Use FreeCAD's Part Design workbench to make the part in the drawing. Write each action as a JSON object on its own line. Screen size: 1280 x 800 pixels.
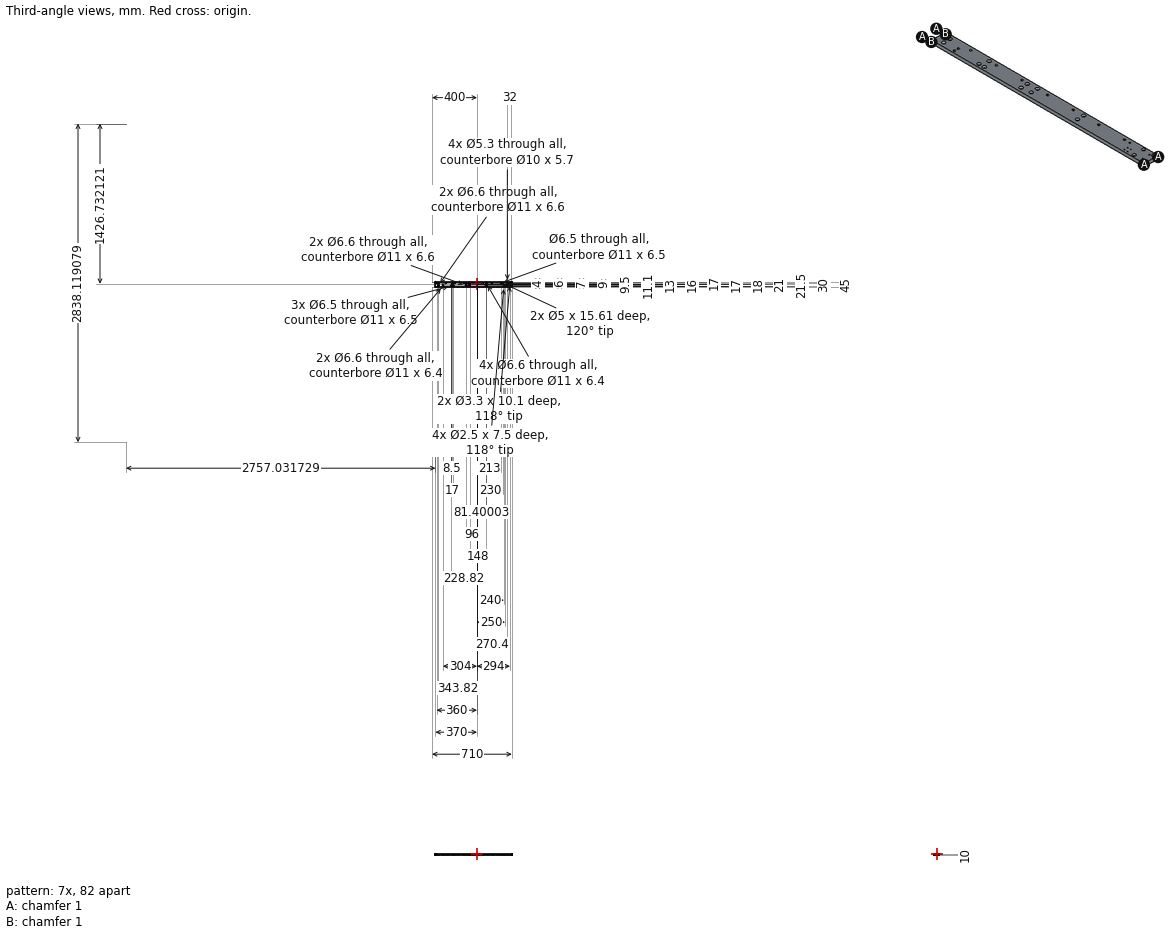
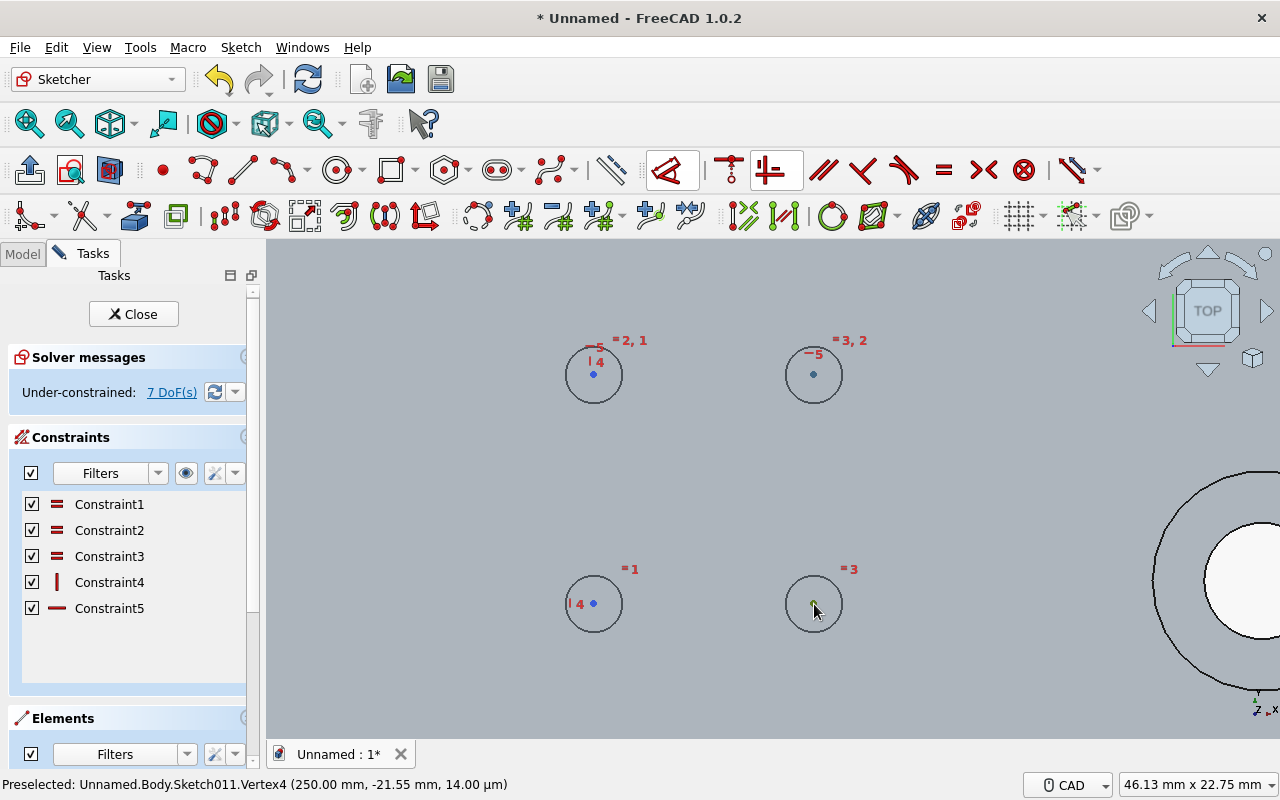
{"action": "left_click", "coordinate": [798, 170]}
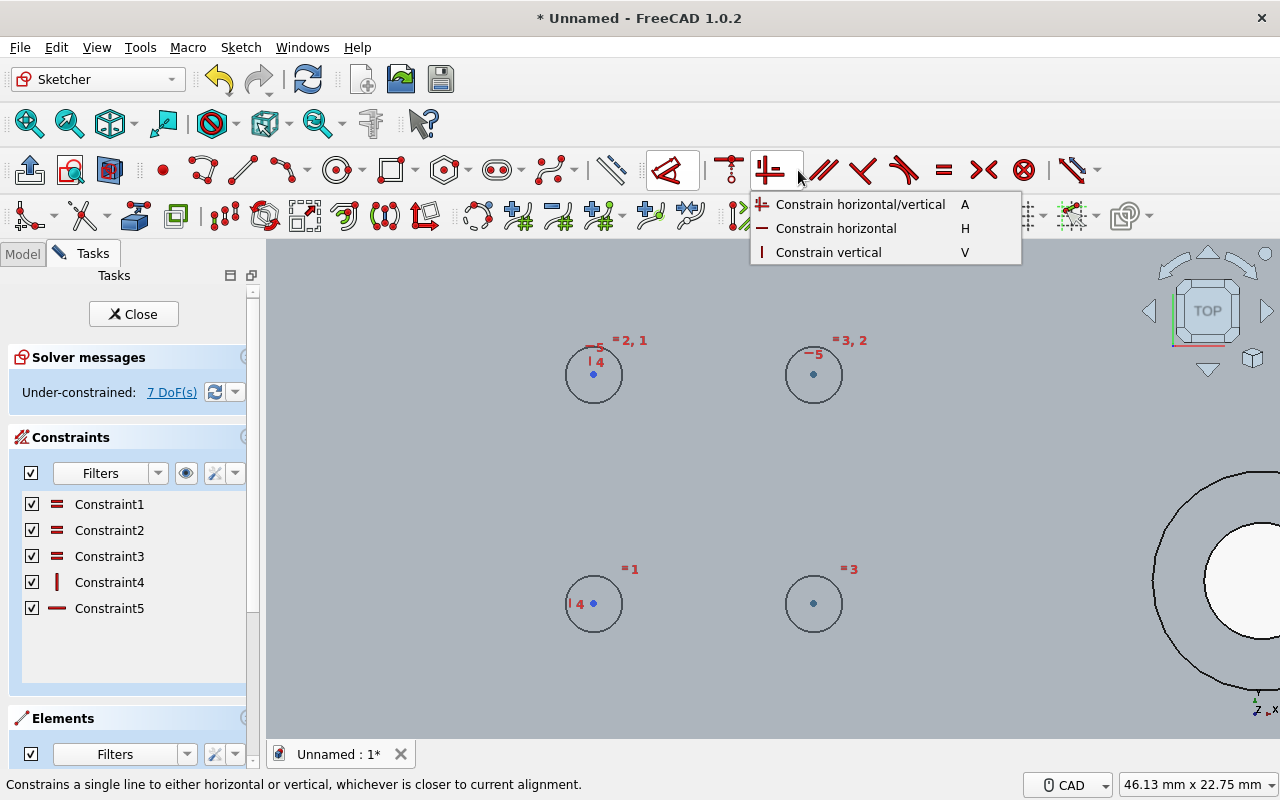
{"action": "left_click", "coordinate": [886, 252]}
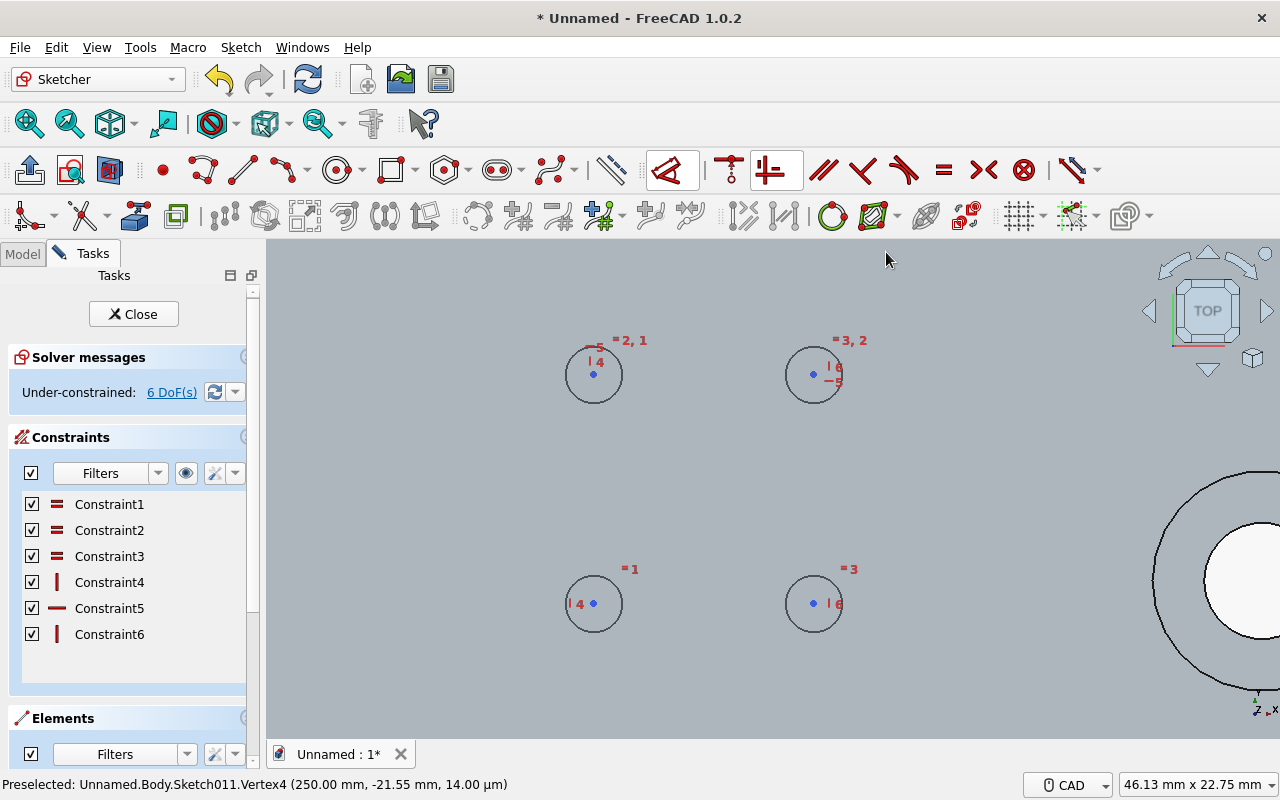
{"action": "left_click", "coordinate": [594, 604]}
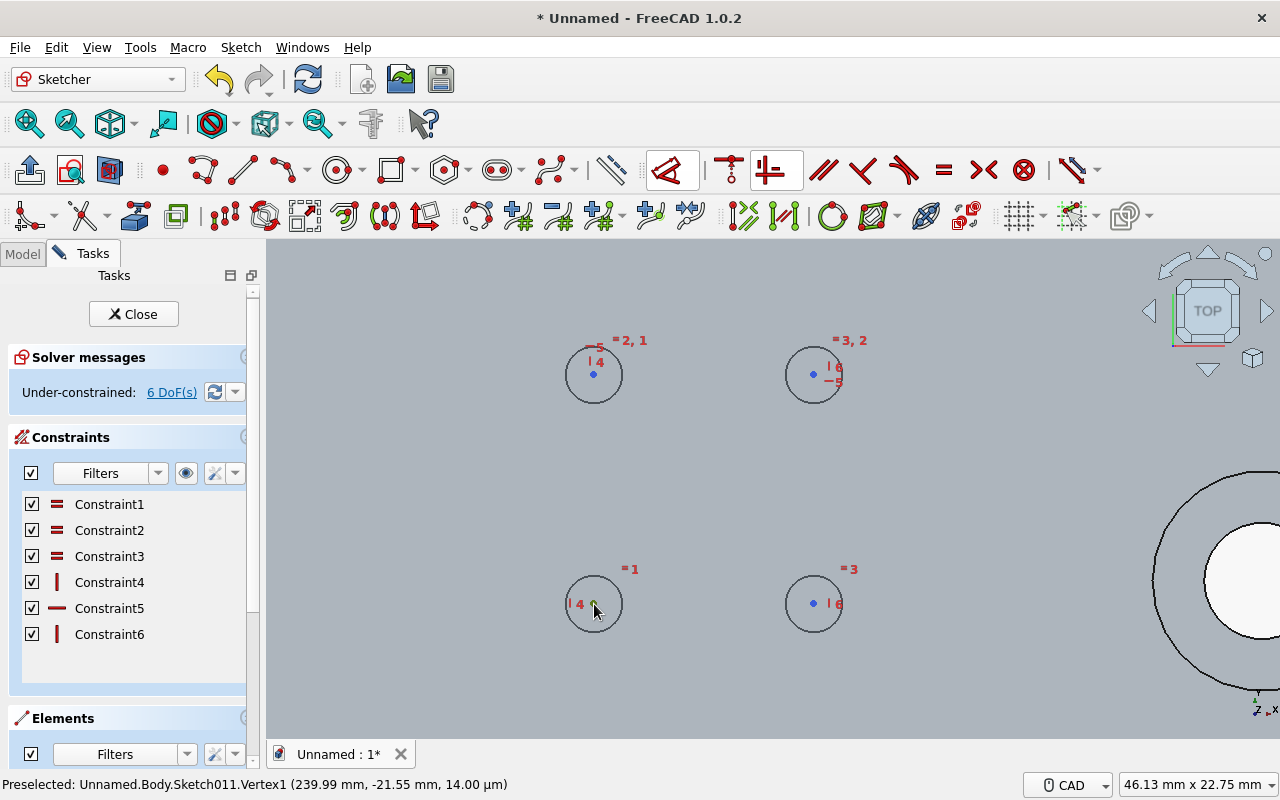
{"action": "left_click", "coordinate": [814, 604]}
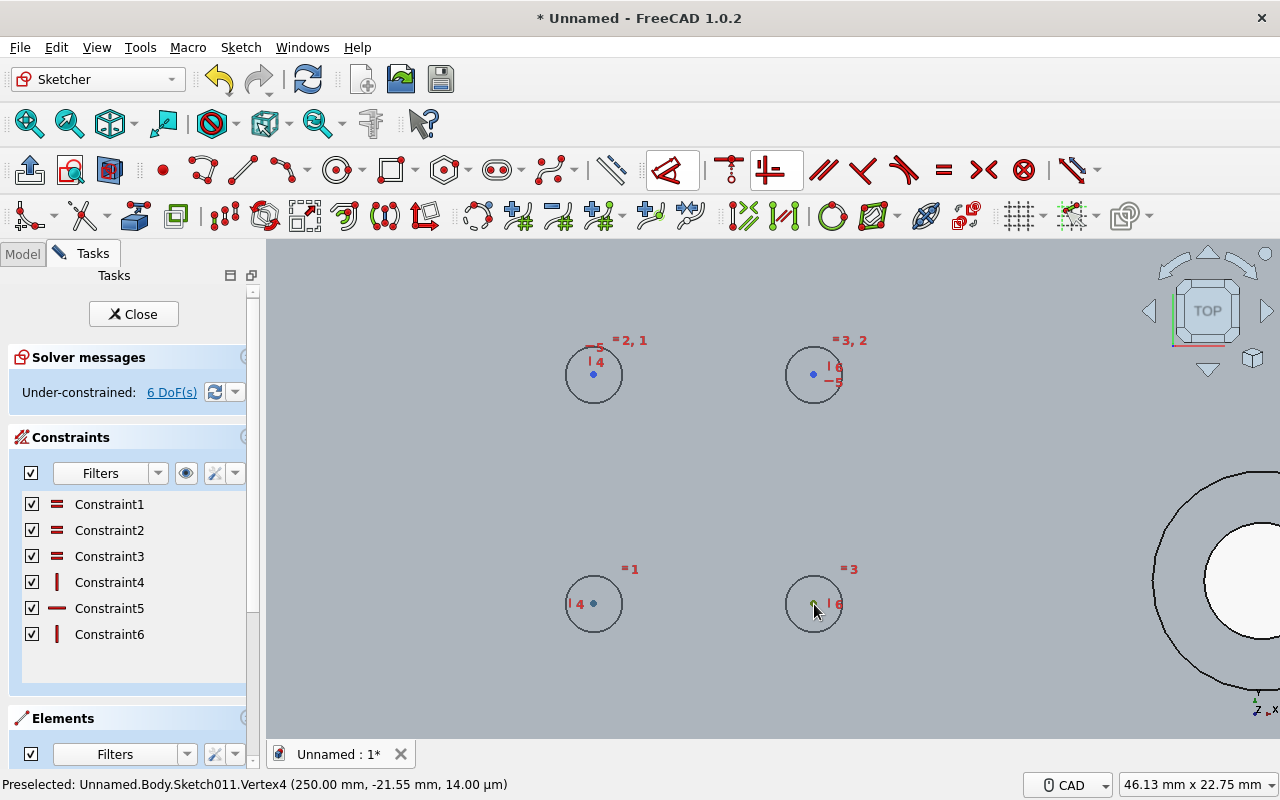
{"action": "key", "text": "h"}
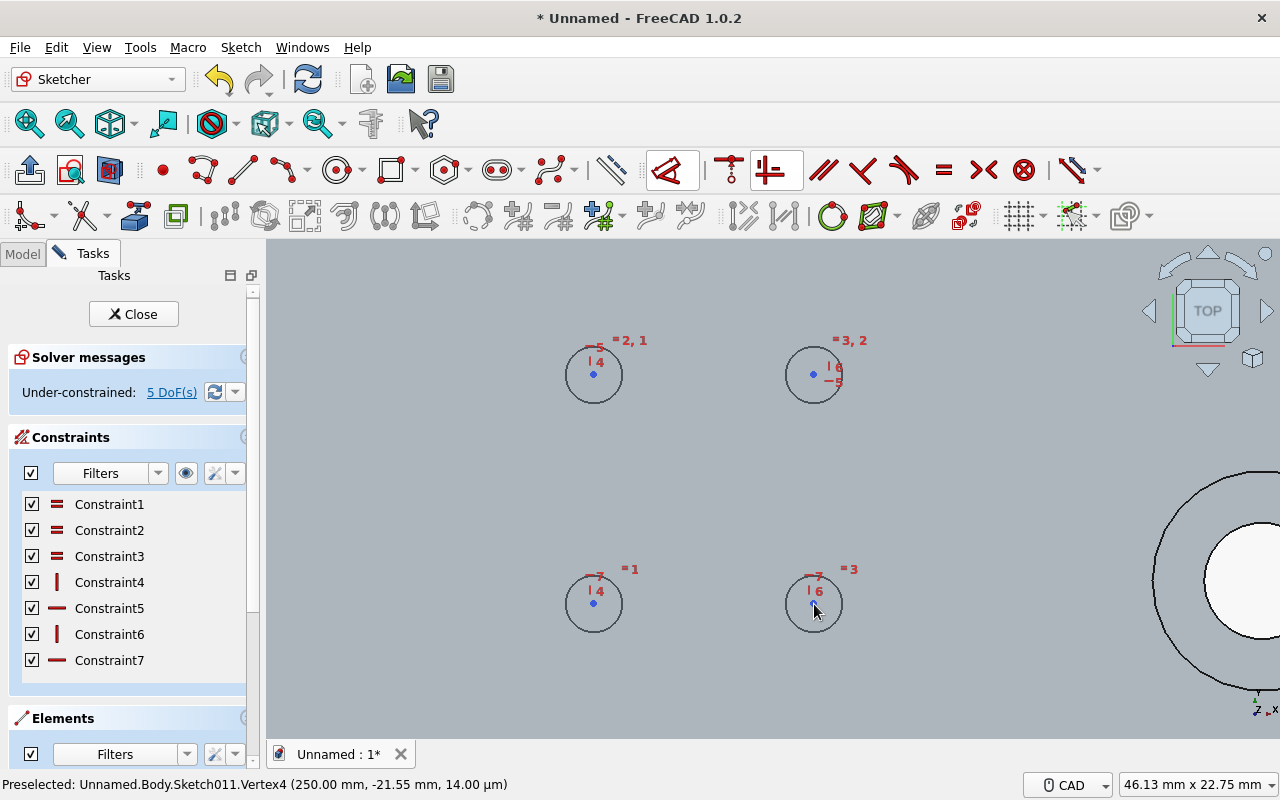
{"action": "left_click", "coordinate": [614, 584]}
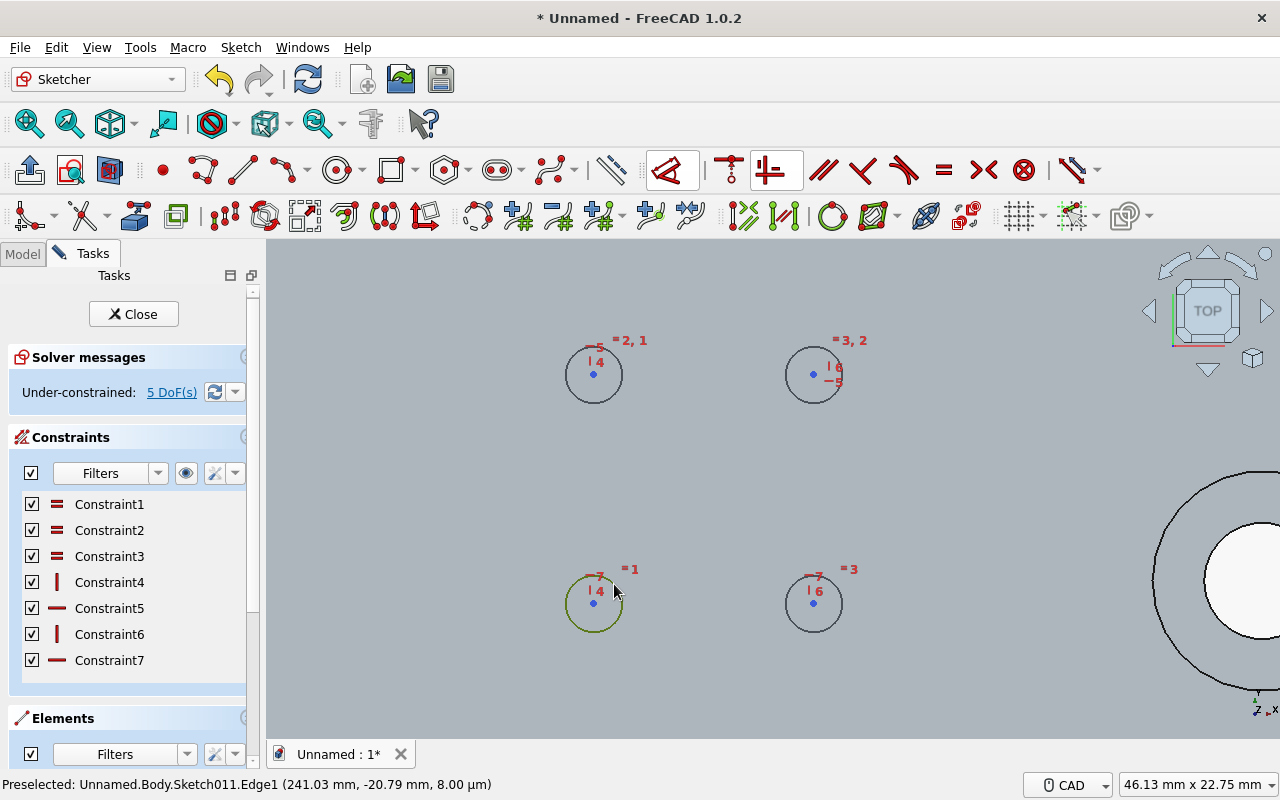
{"action": "key", "text": "k o"}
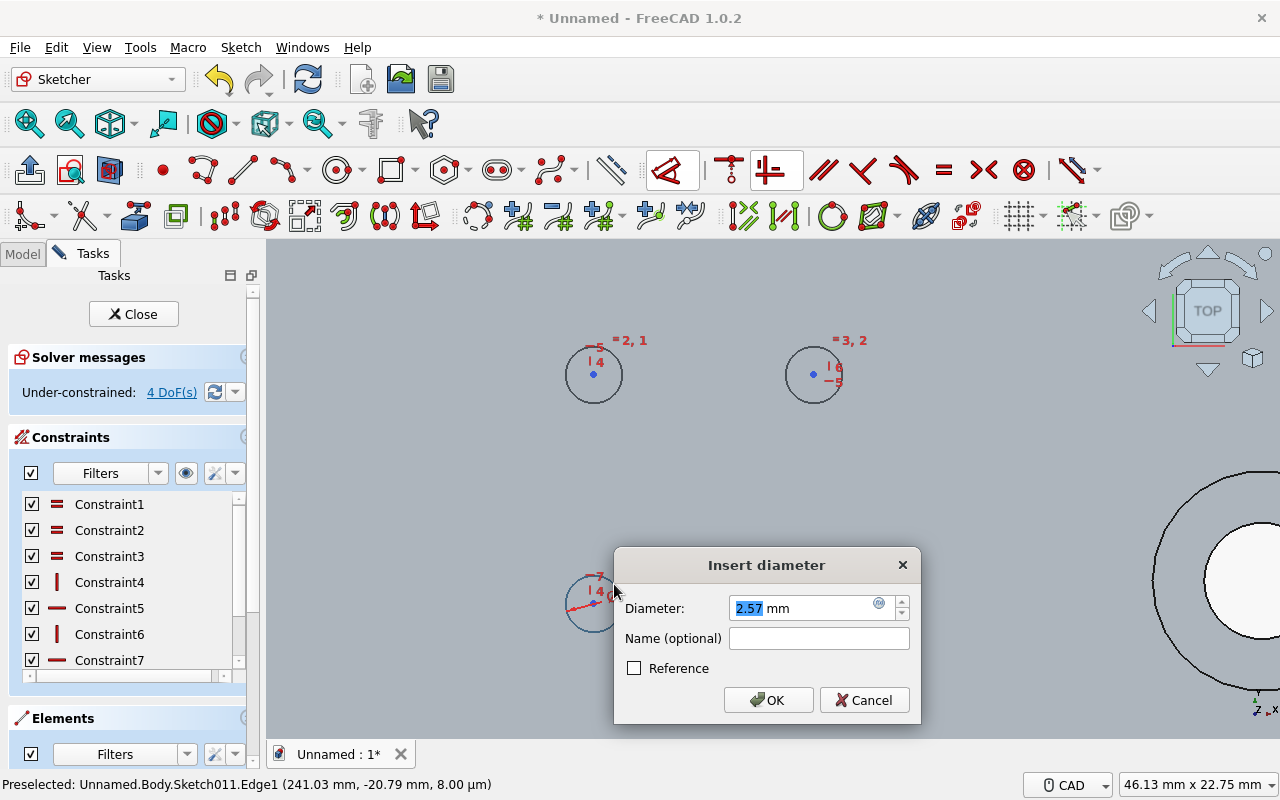
{"action": "type", "text": "2.5"}
{"action": "key", "text": "Return"}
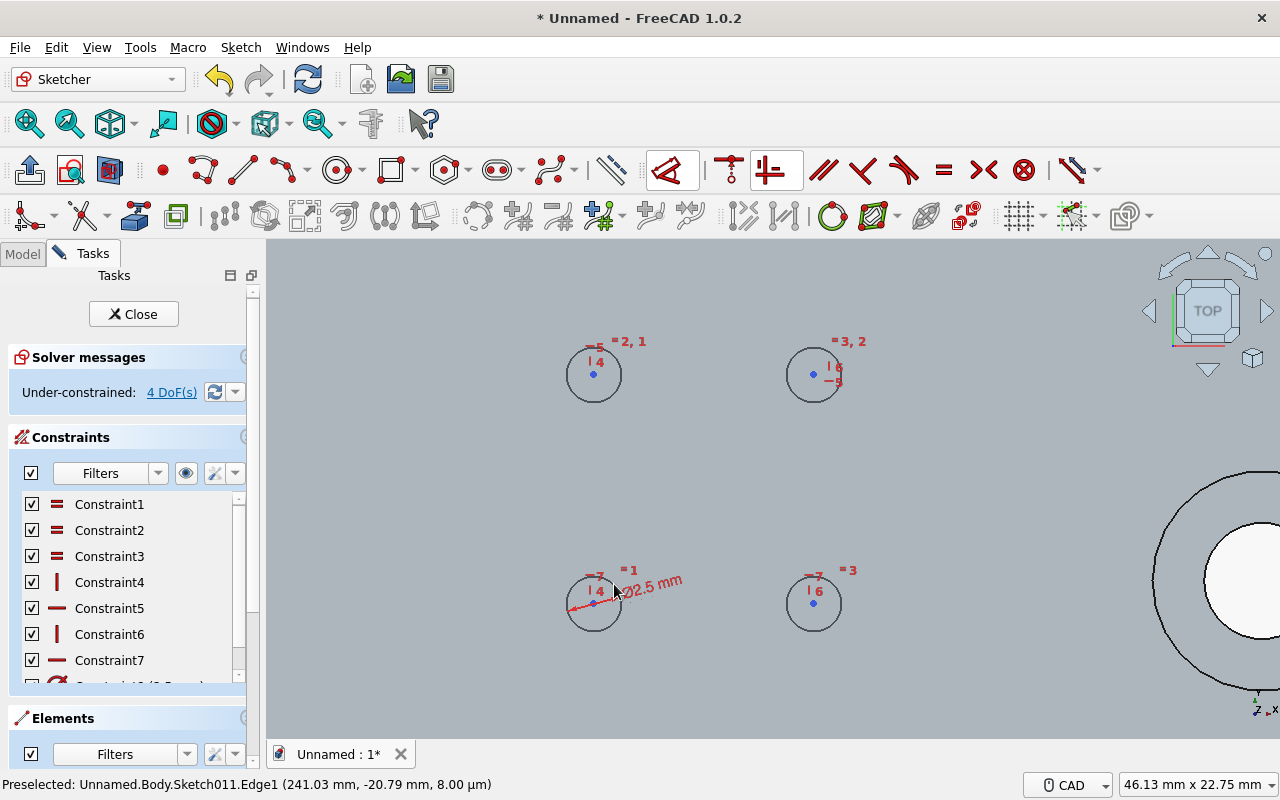
{"action": "left_click", "coordinate": [594, 604]}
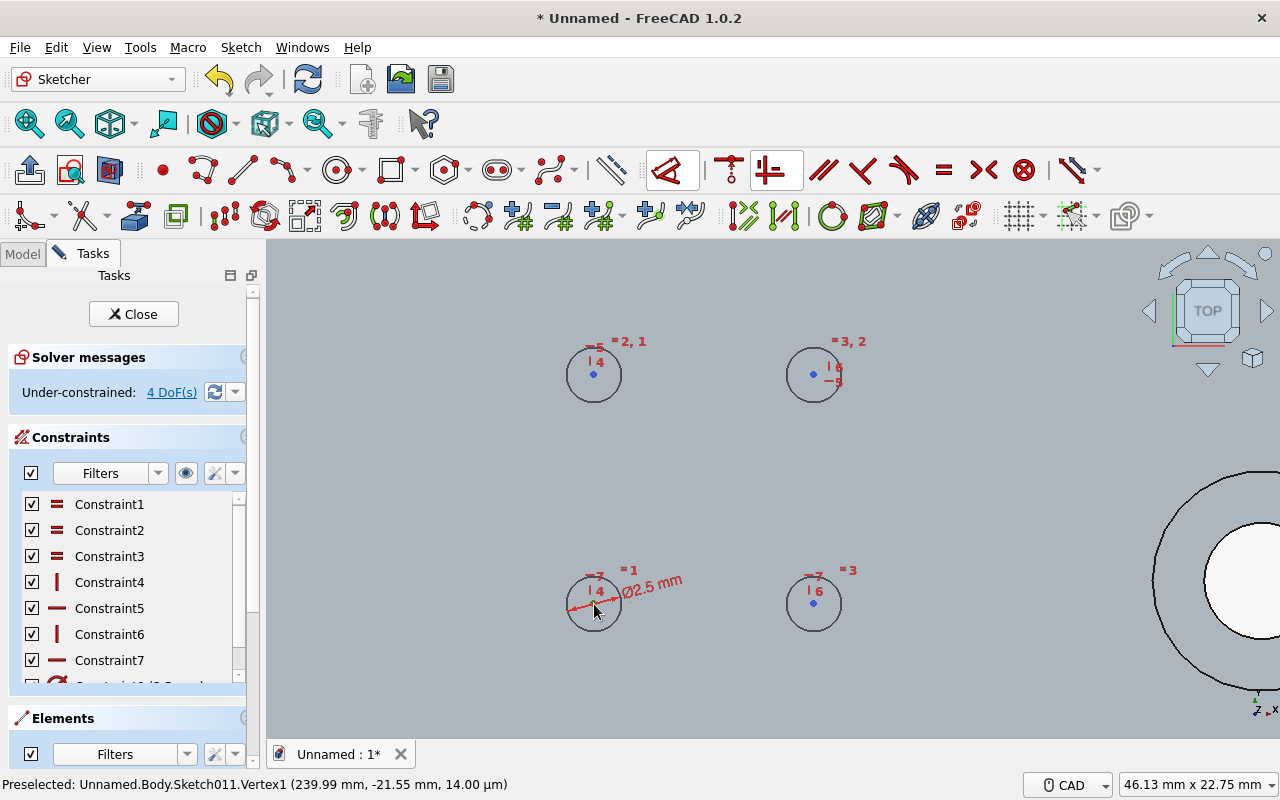
{"action": "left_click", "coordinate": [694, 170]}